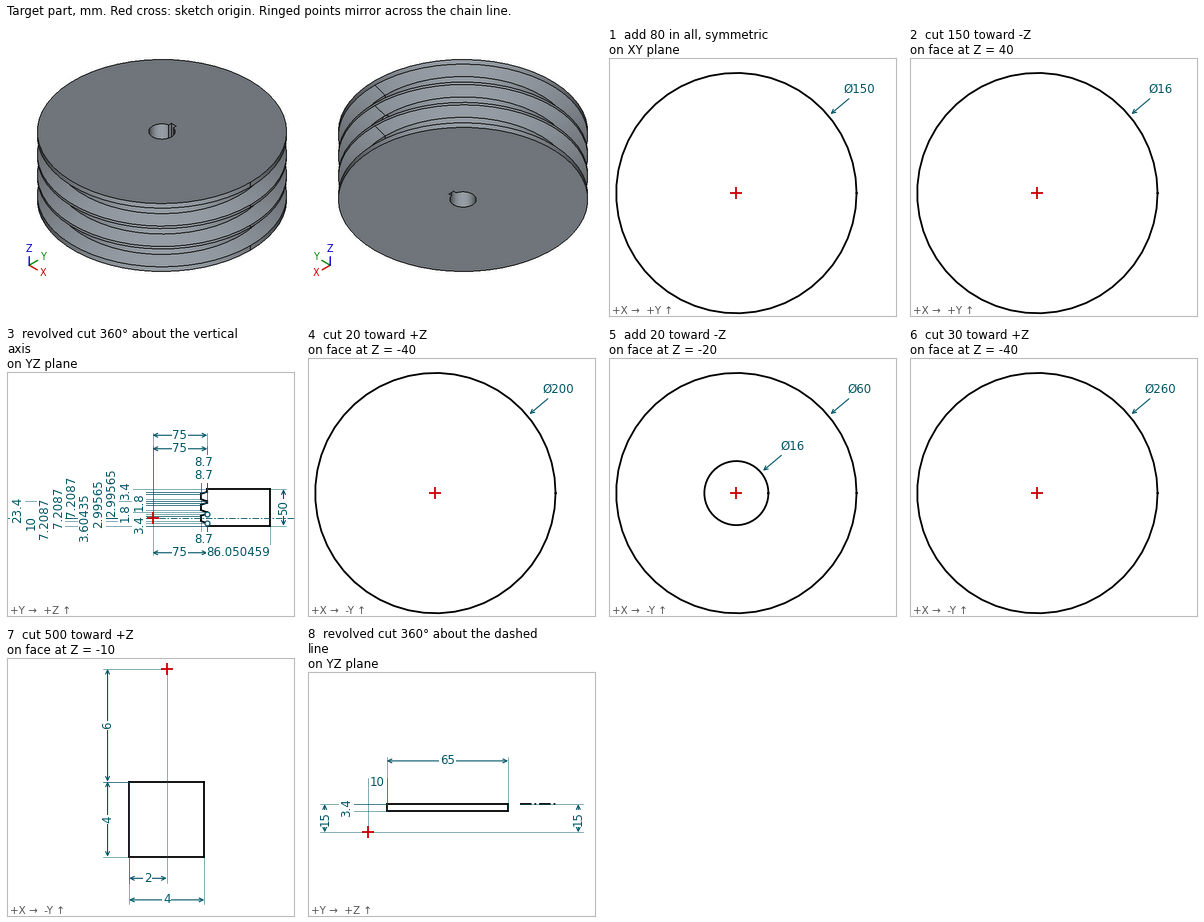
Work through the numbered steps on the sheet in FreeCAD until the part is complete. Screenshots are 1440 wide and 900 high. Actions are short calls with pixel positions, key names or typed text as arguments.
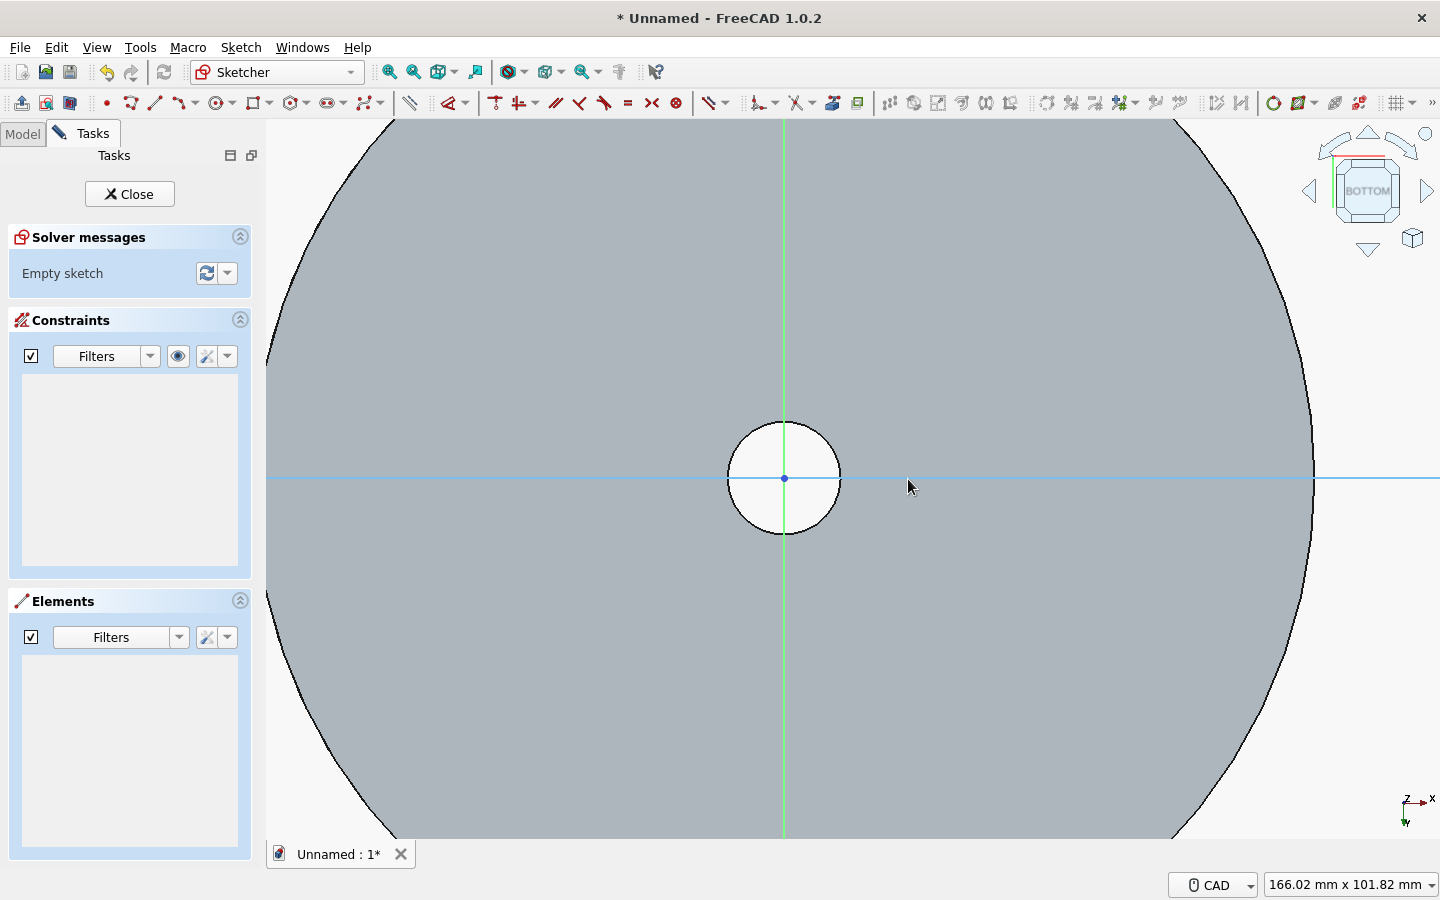
key(g)
key(c)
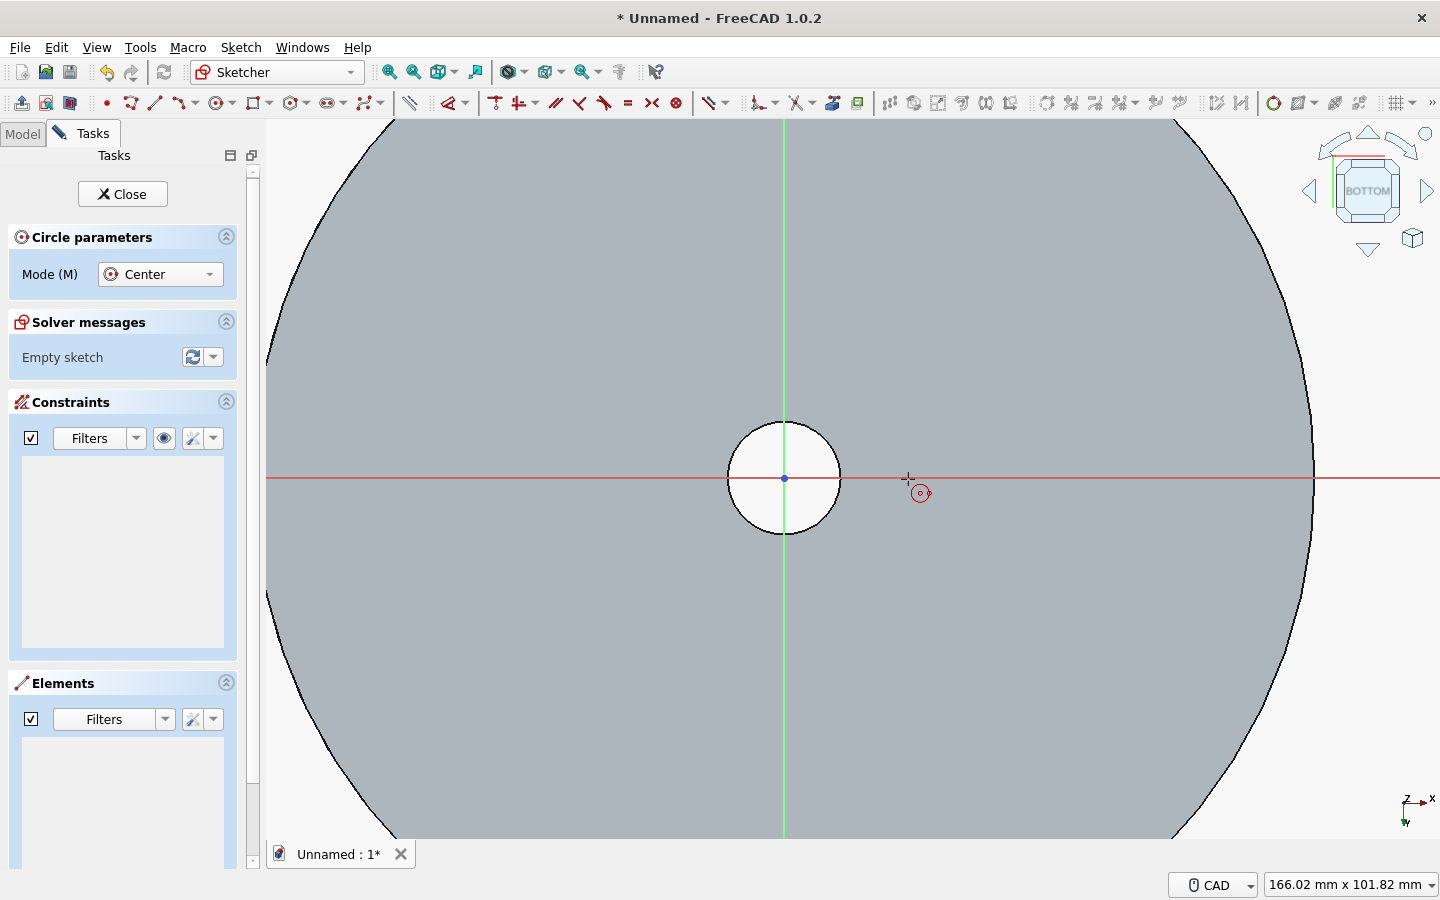
click(784, 478)
click(934, 328)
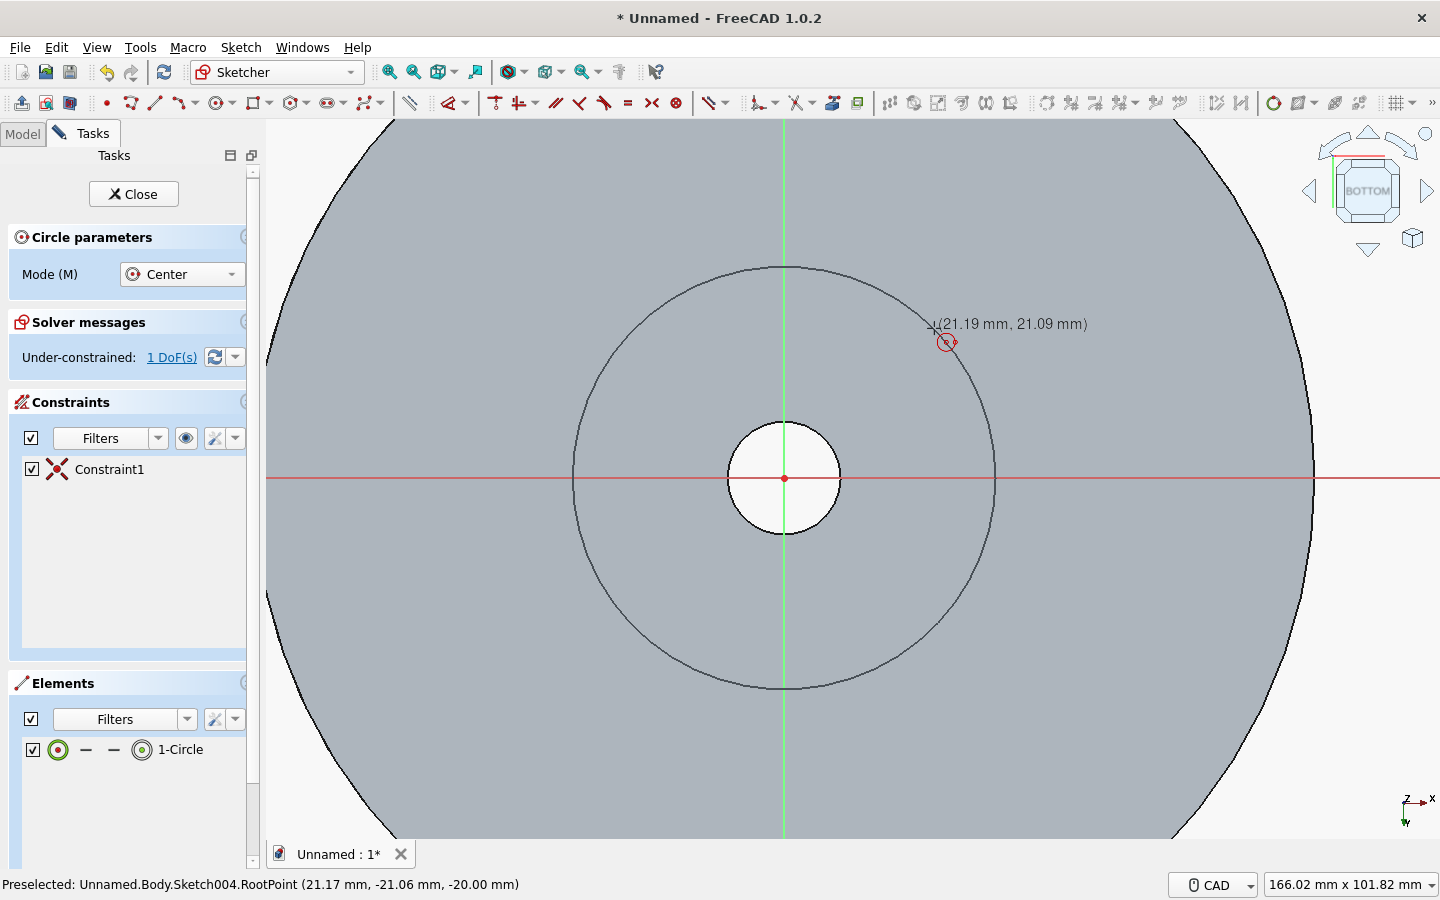
click(784, 478)
click(824, 438)
key(Escape)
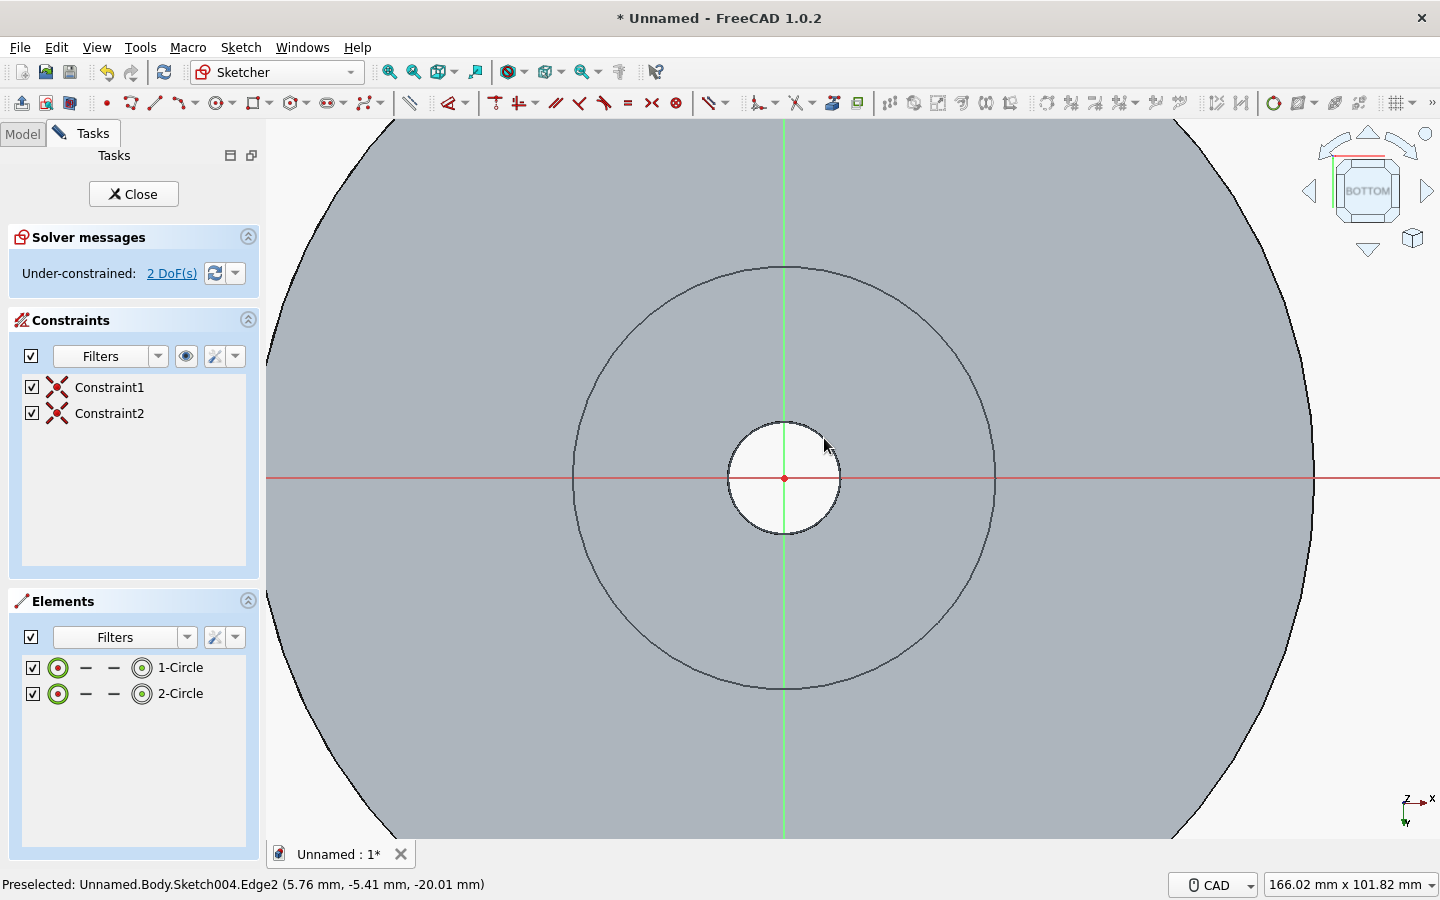
click(448, 104)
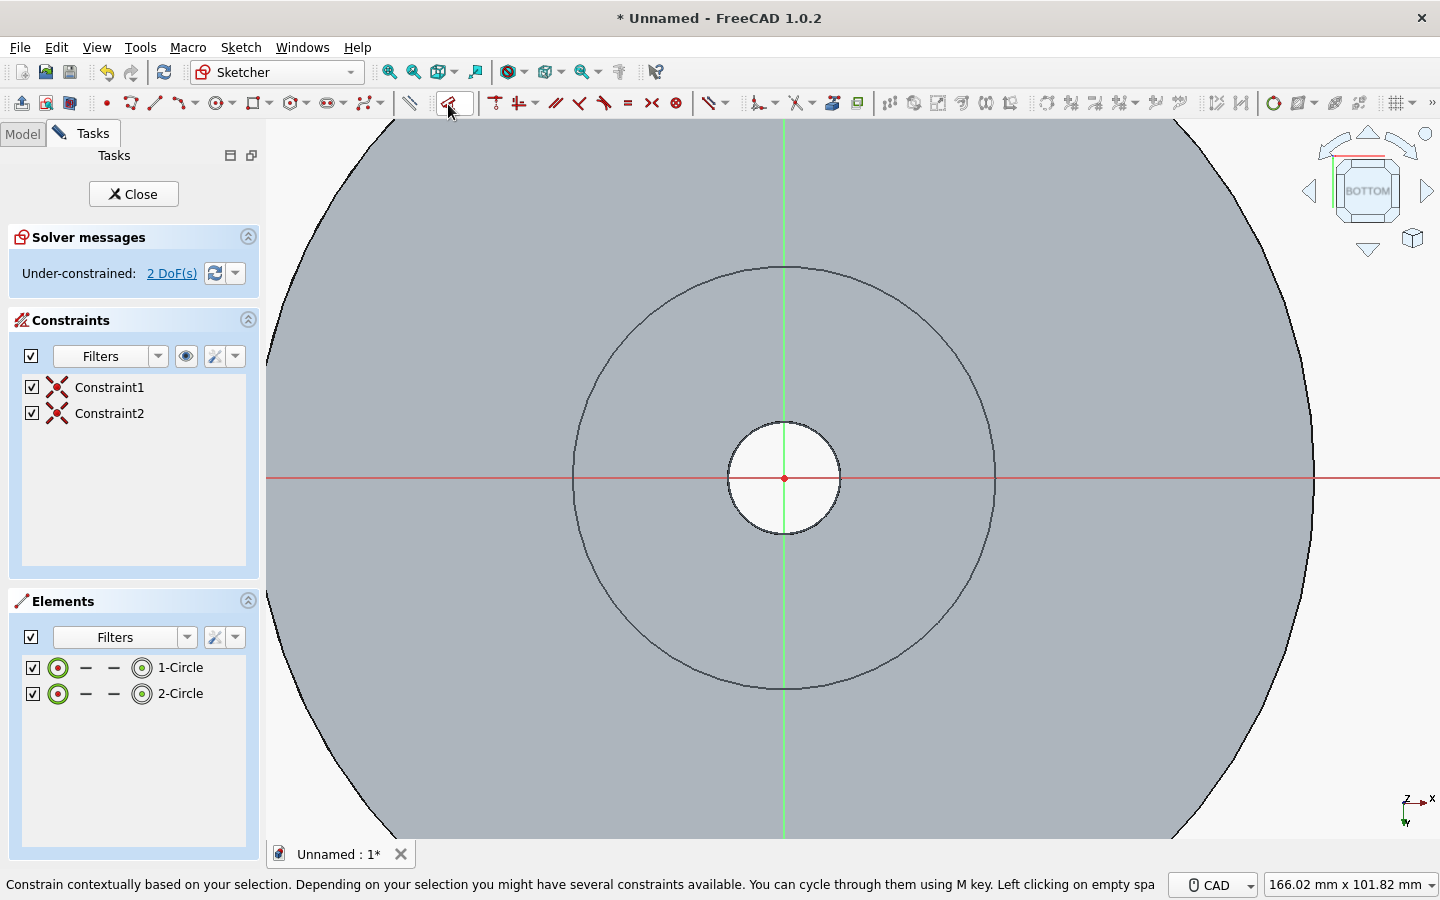
click(933, 328)
click(956, 305)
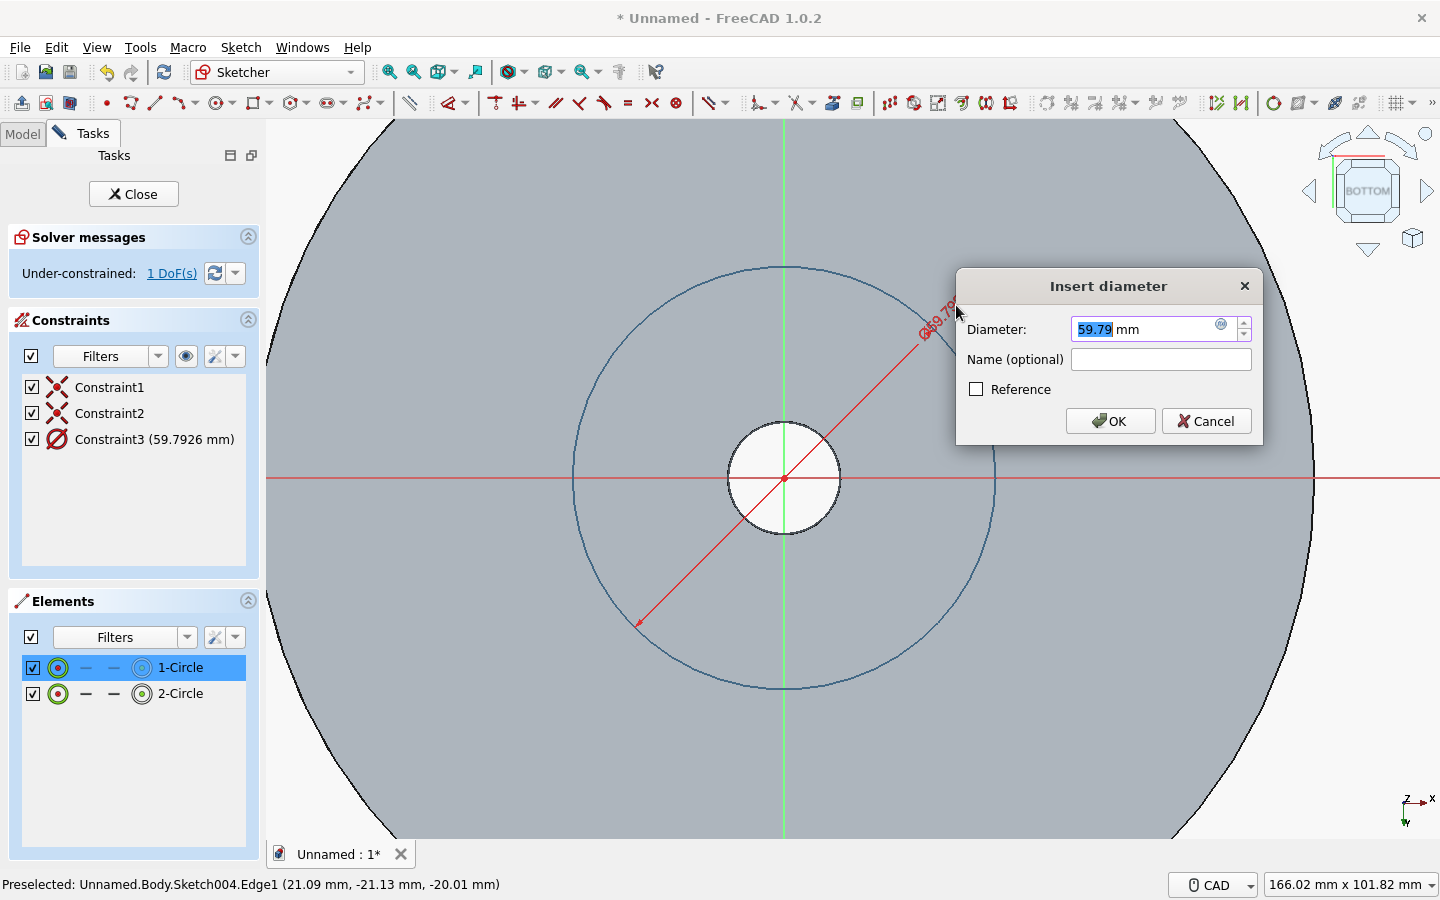
text(60)
key(Return)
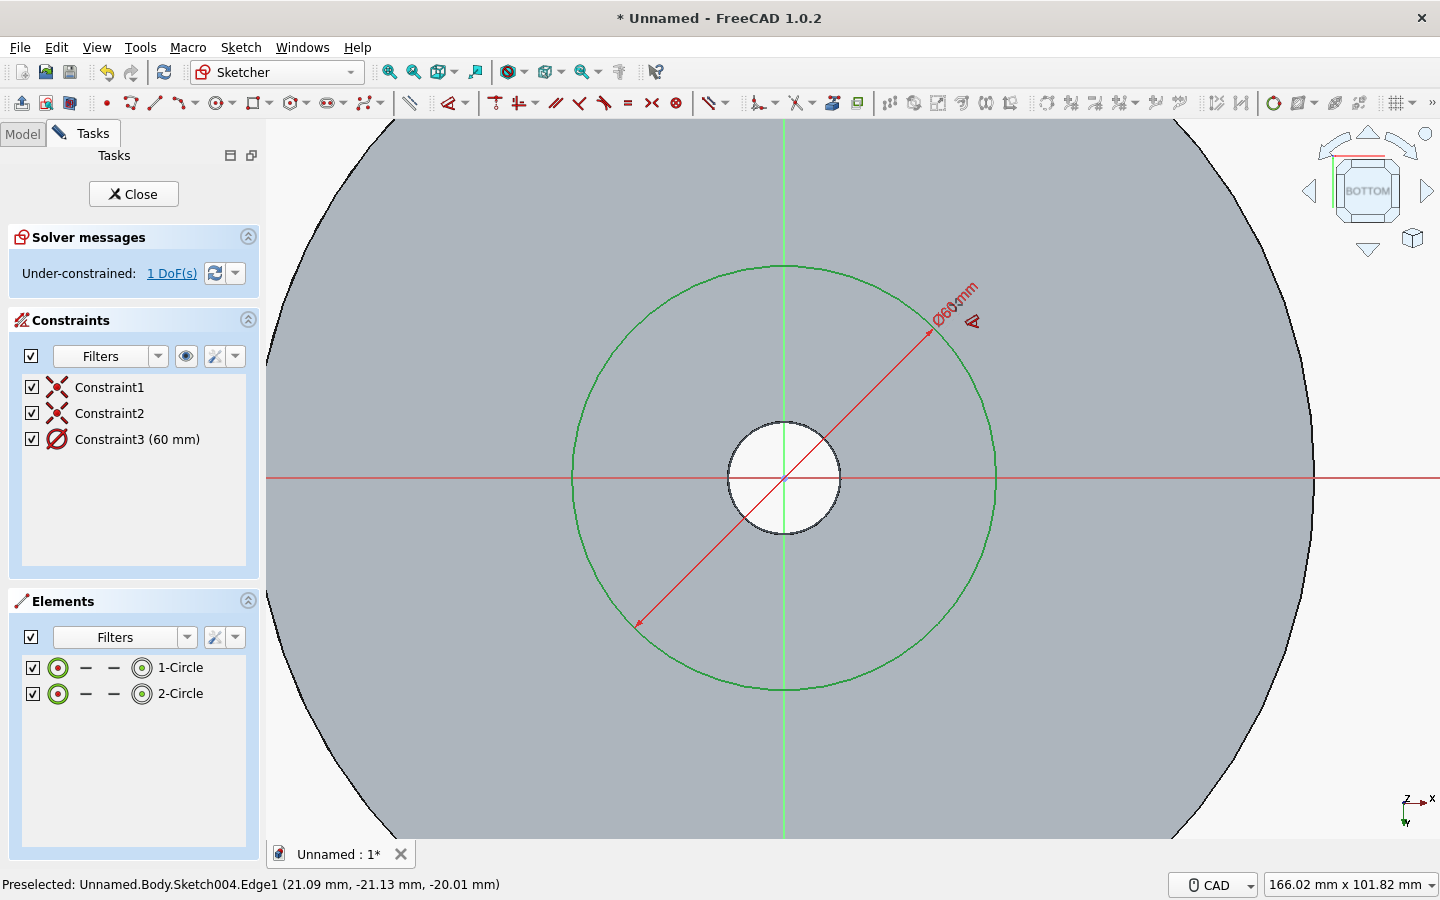
click(823, 438)
click(845, 415)